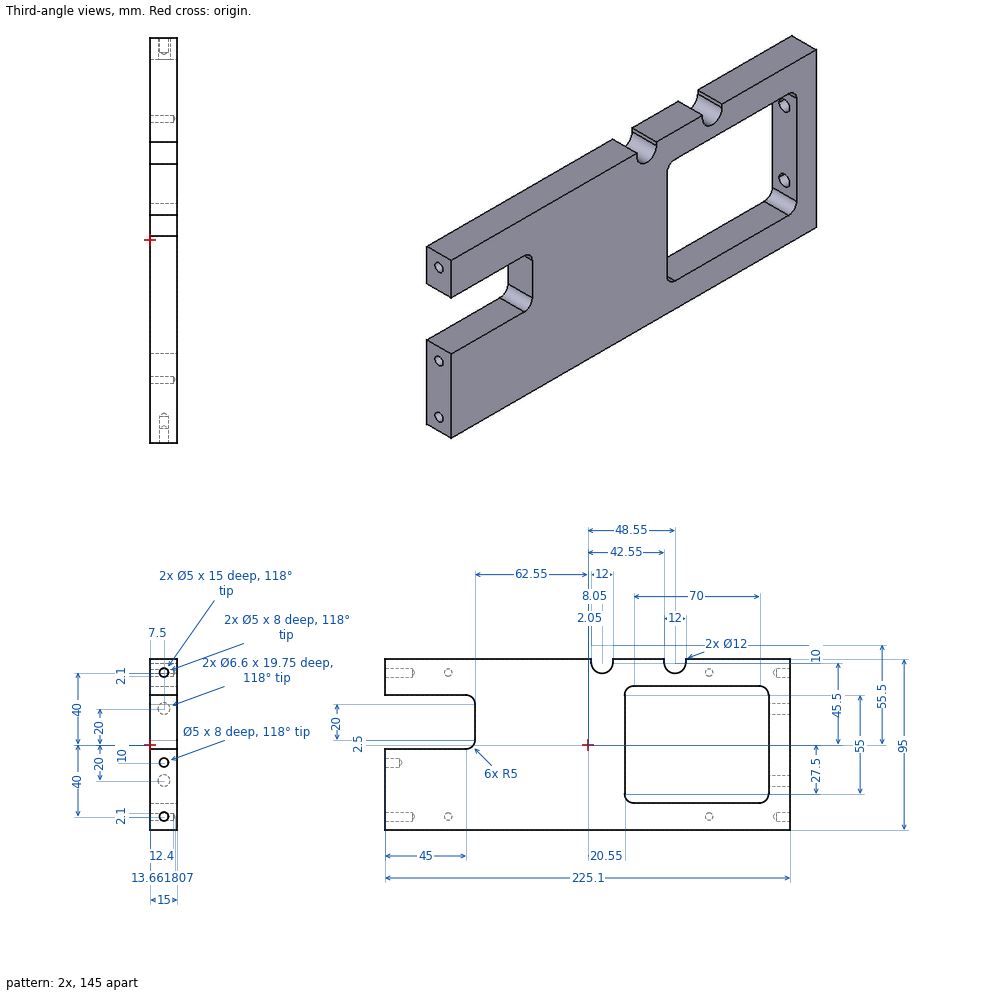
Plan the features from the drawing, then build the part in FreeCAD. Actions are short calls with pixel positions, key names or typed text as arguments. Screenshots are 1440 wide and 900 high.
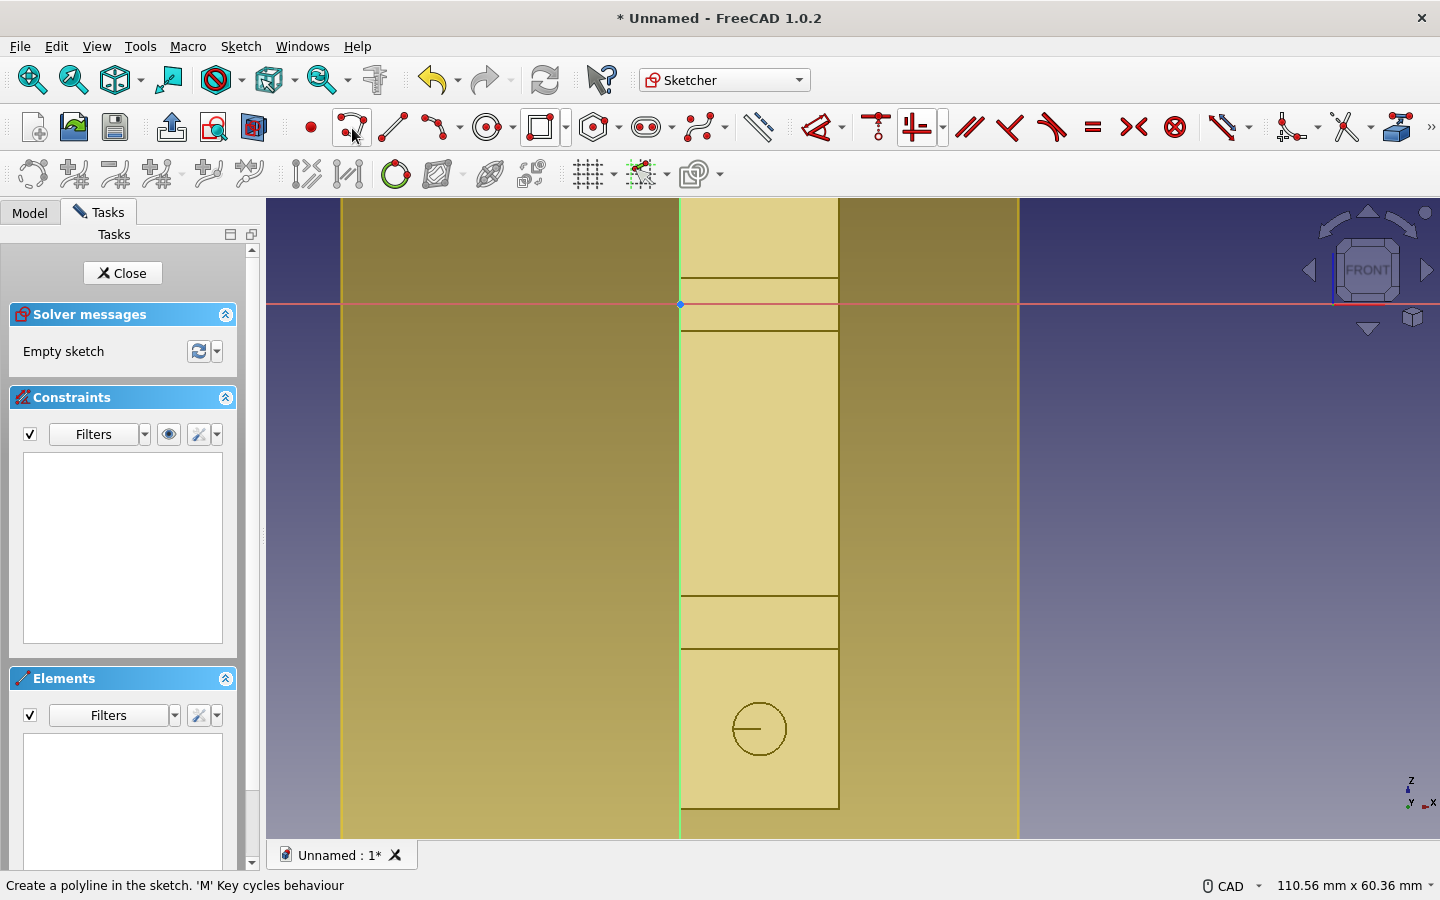
click(680, 707)
click(812, 707)
click(825, 729)
click(689, 729)
click(680, 708)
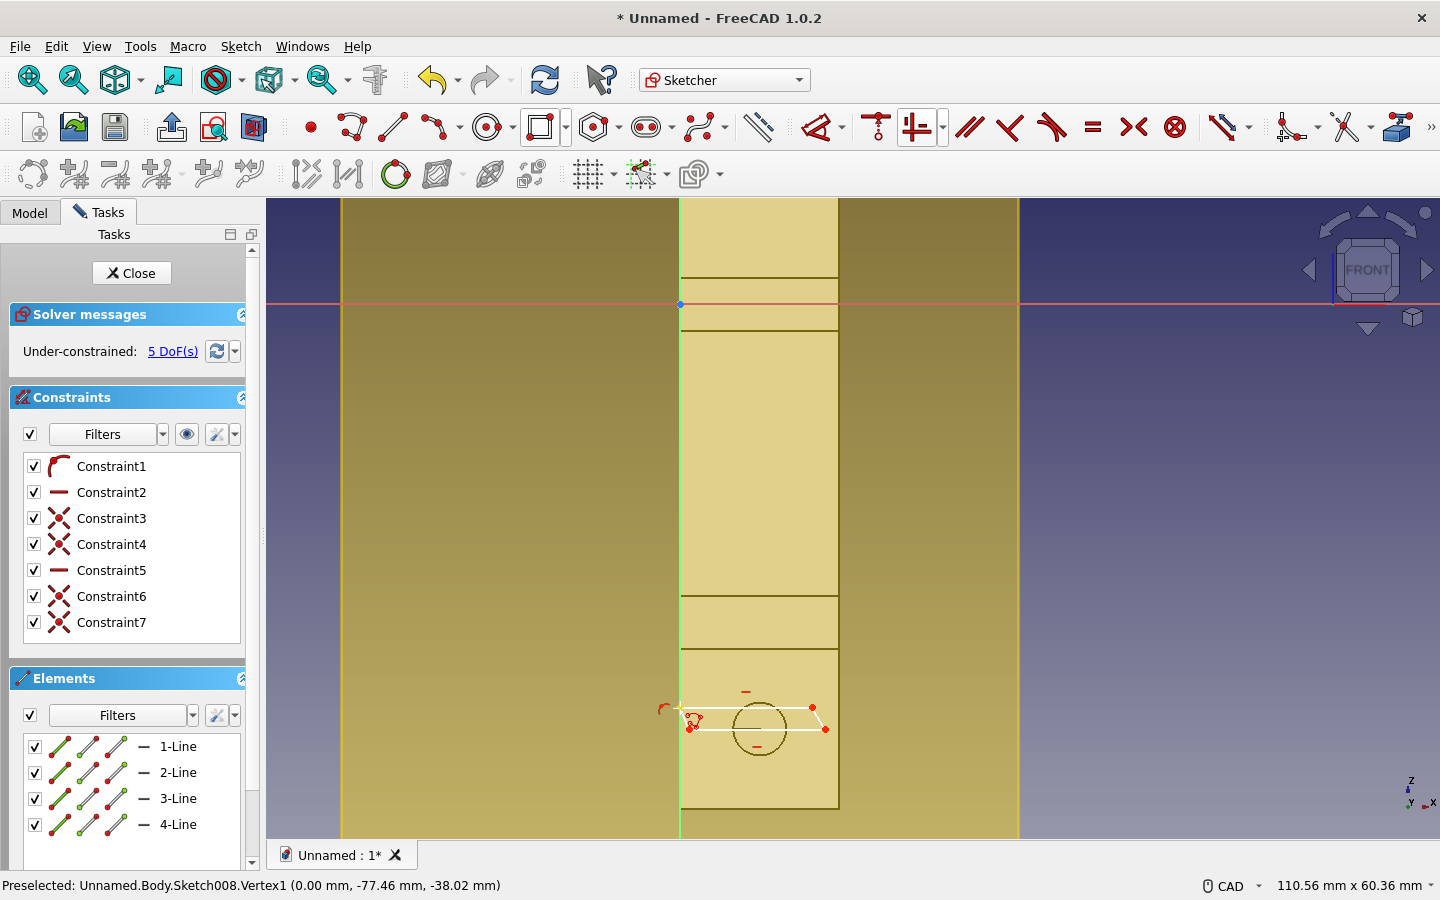
click(393, 128)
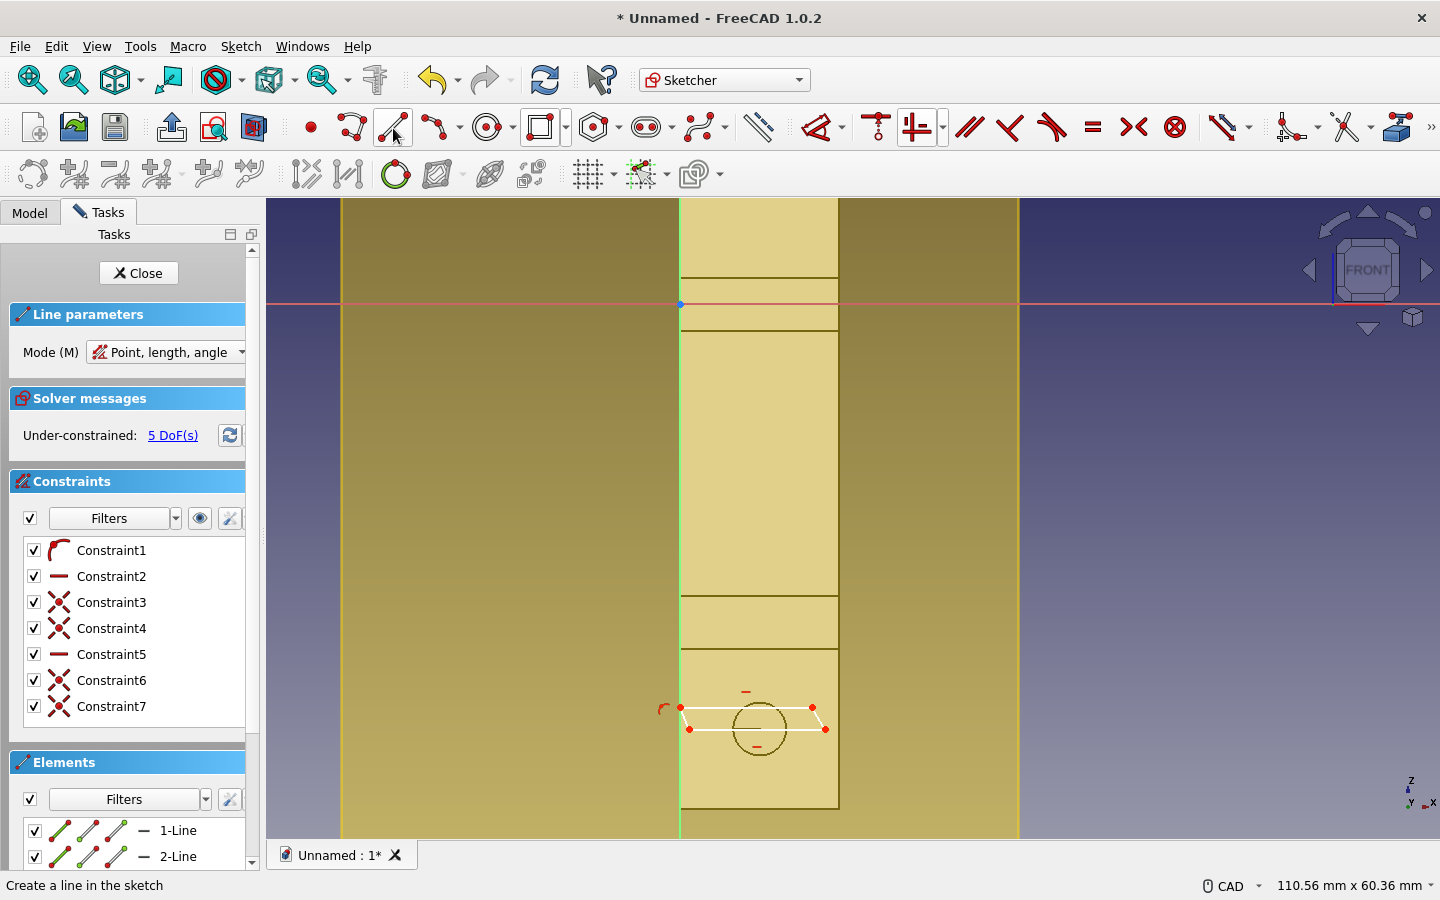
click(840, 729)
click(883, 729)
key(Escape)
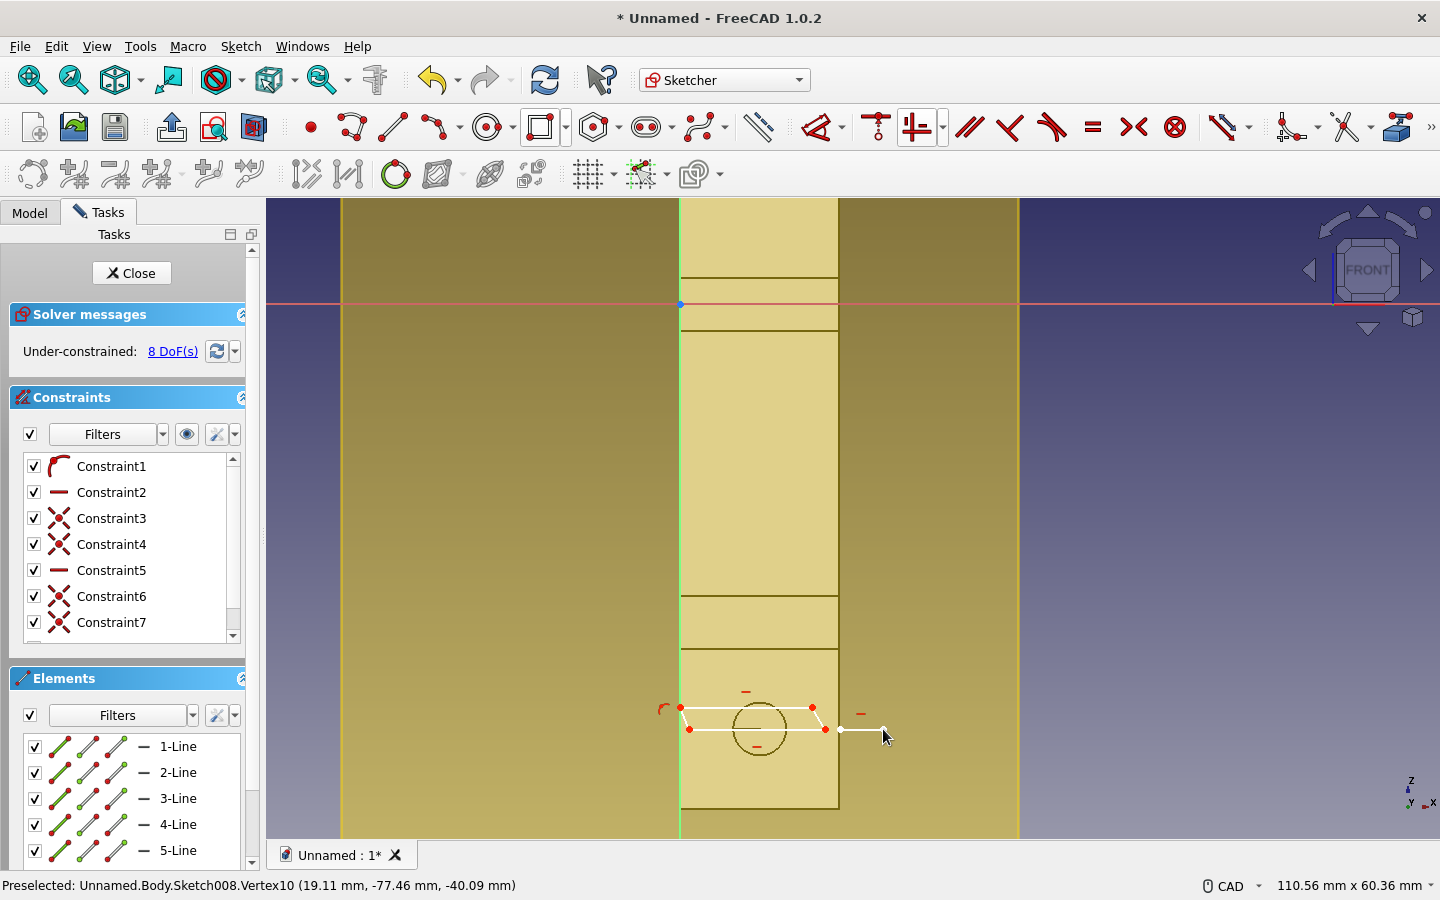
click(853, 730)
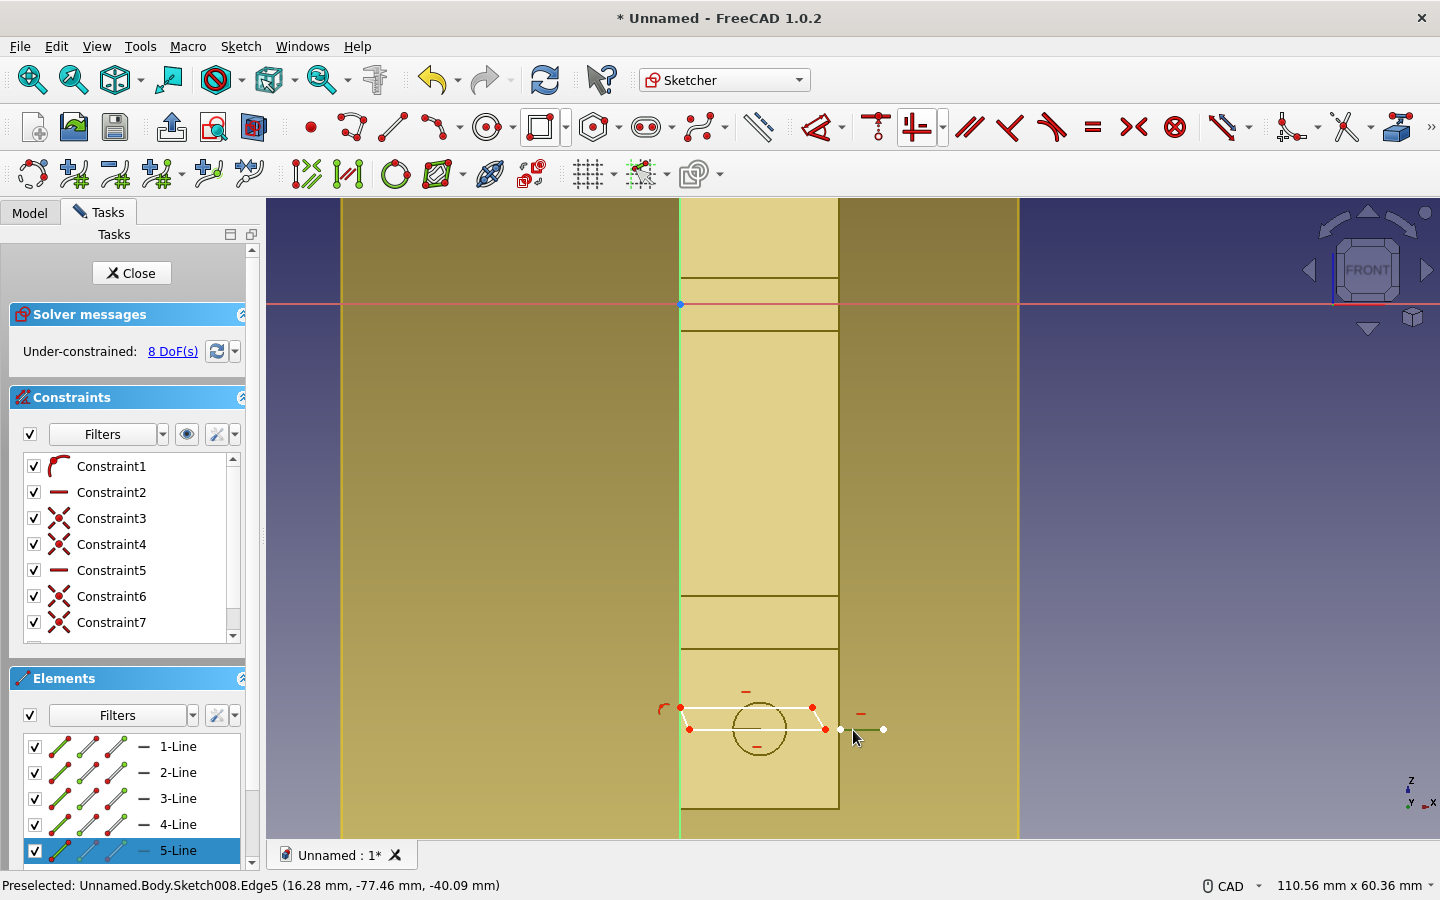
click(759, 128)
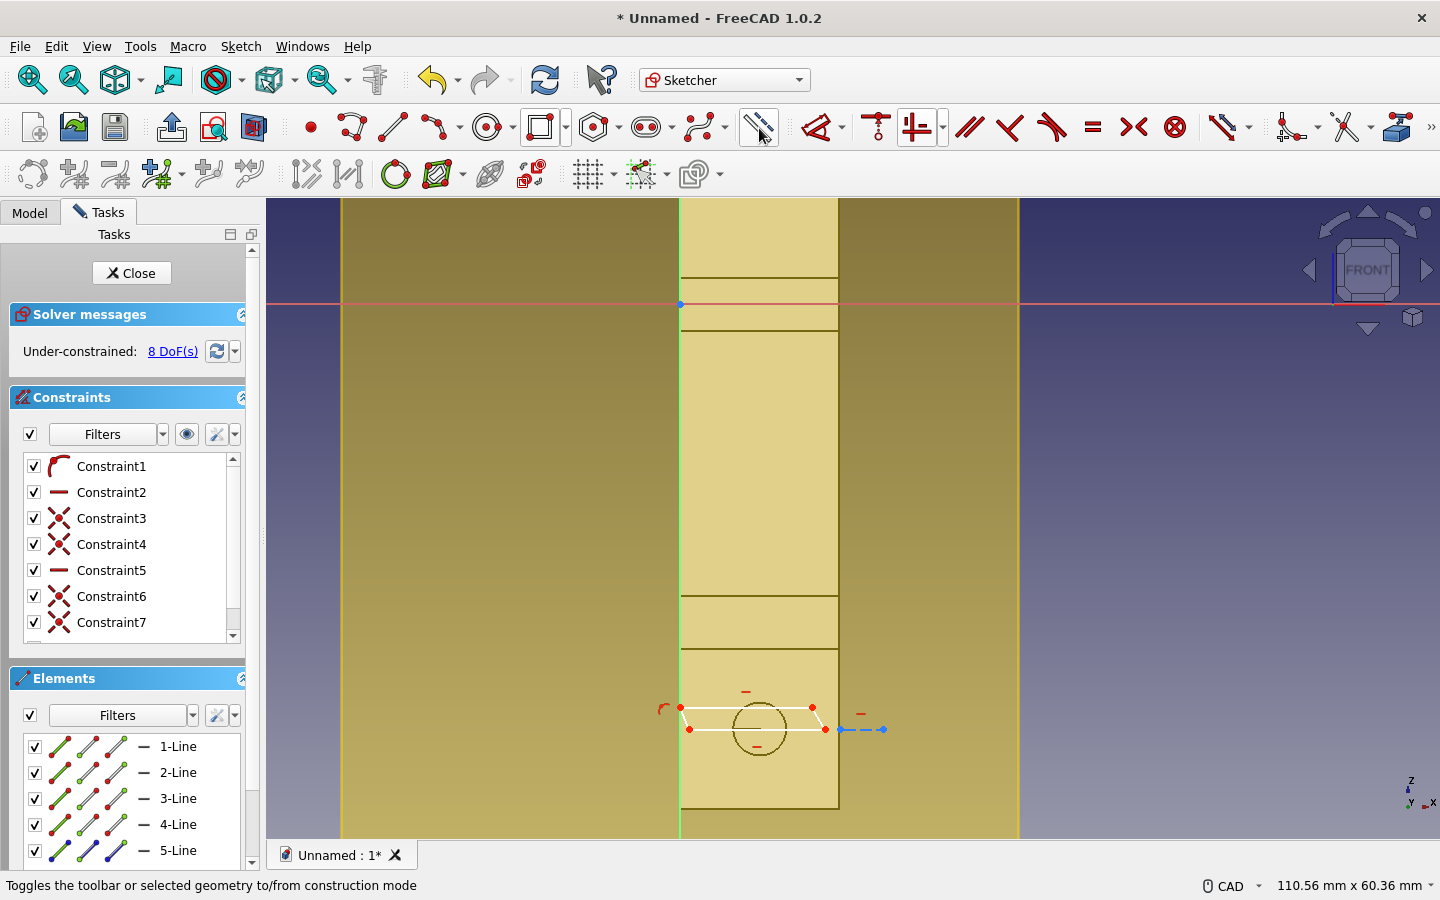
scroll(684, 717, up, 3)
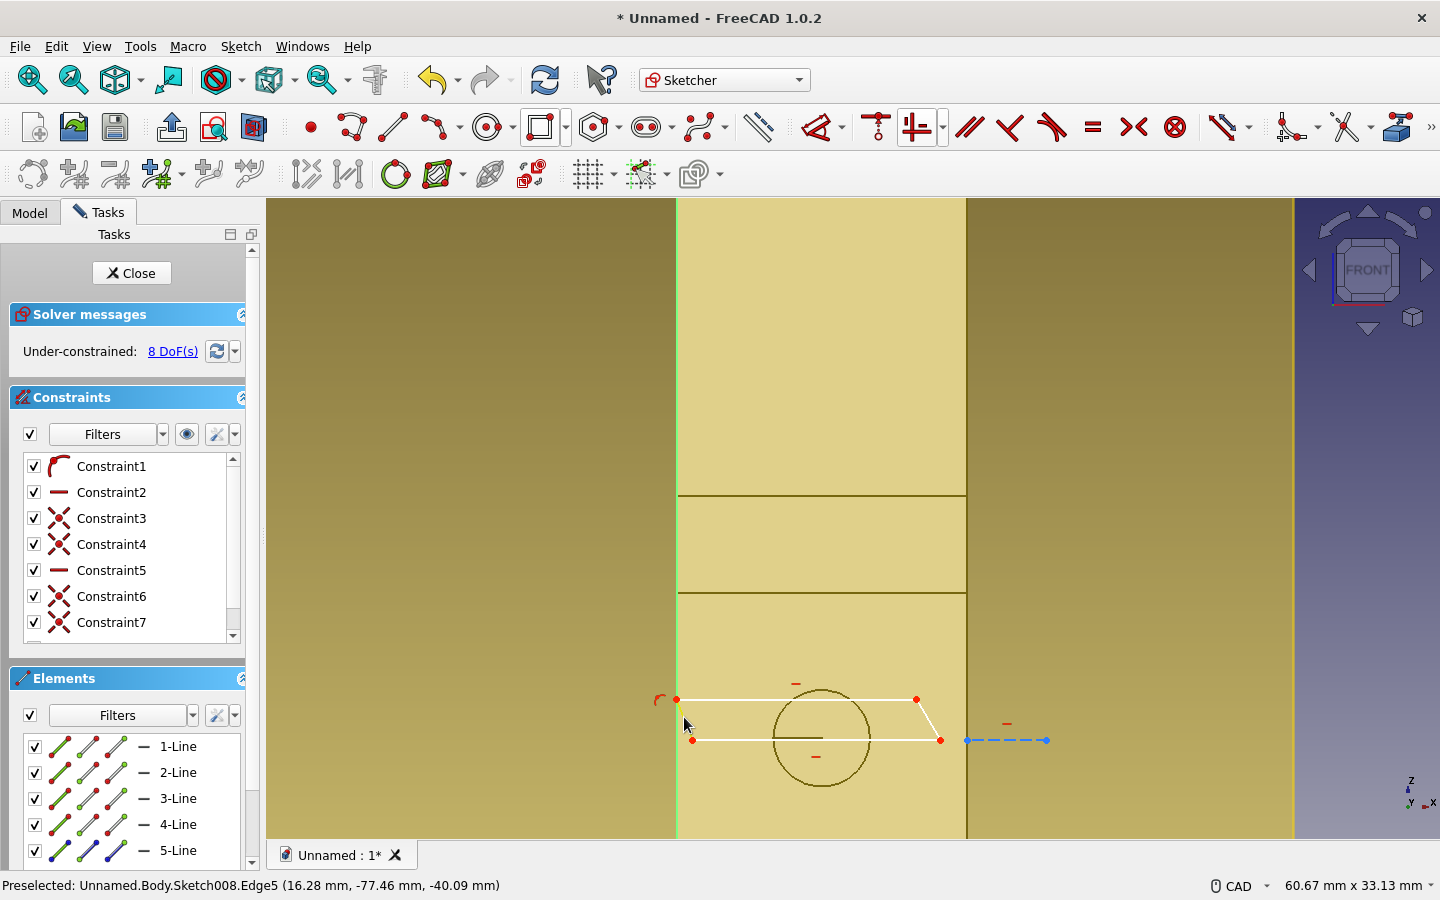
click(683, 716)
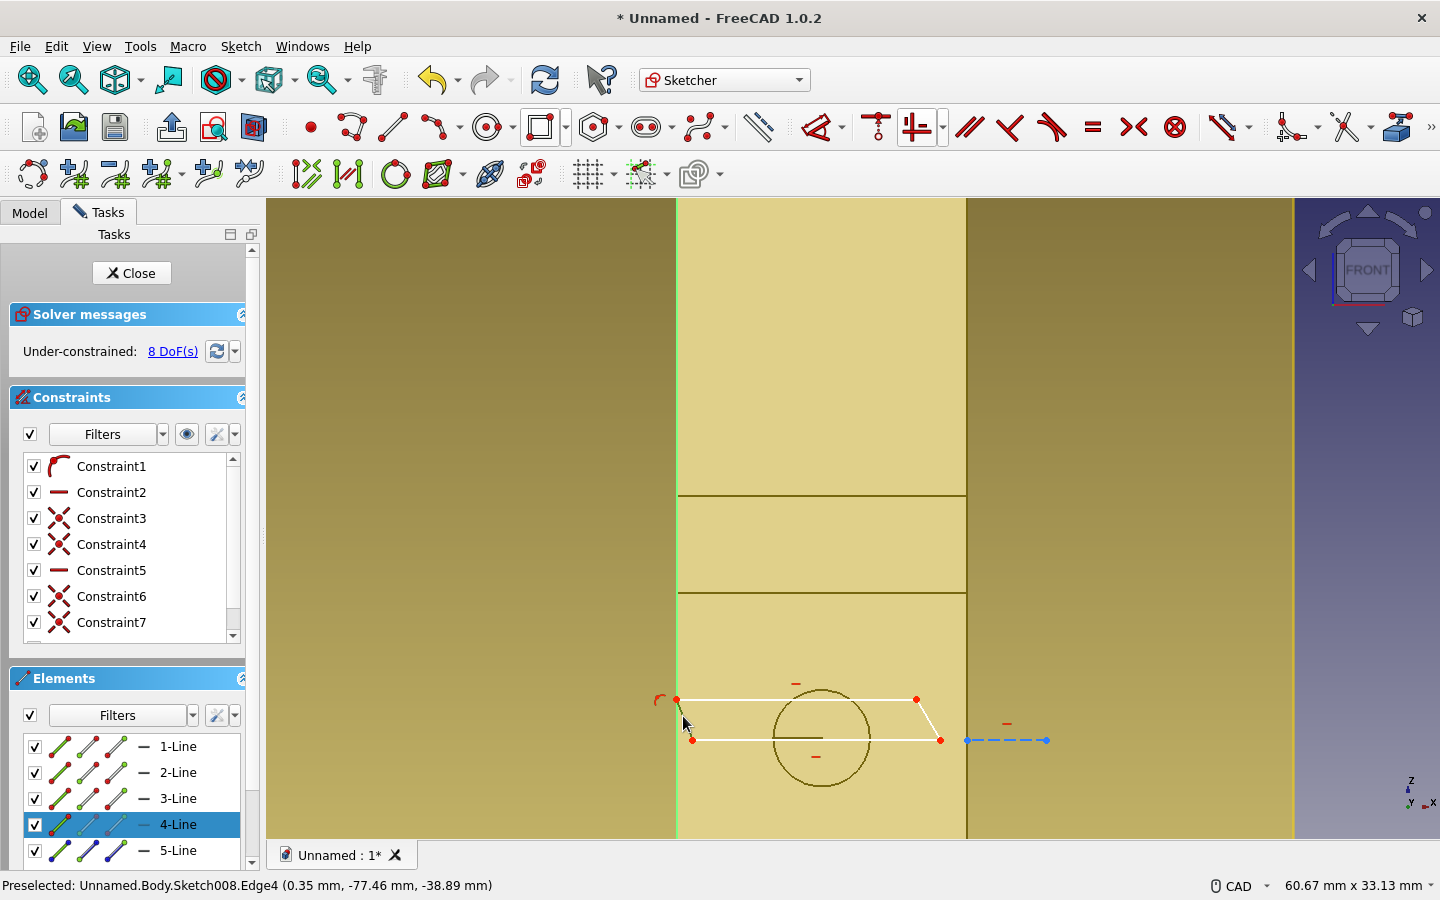
key(v)